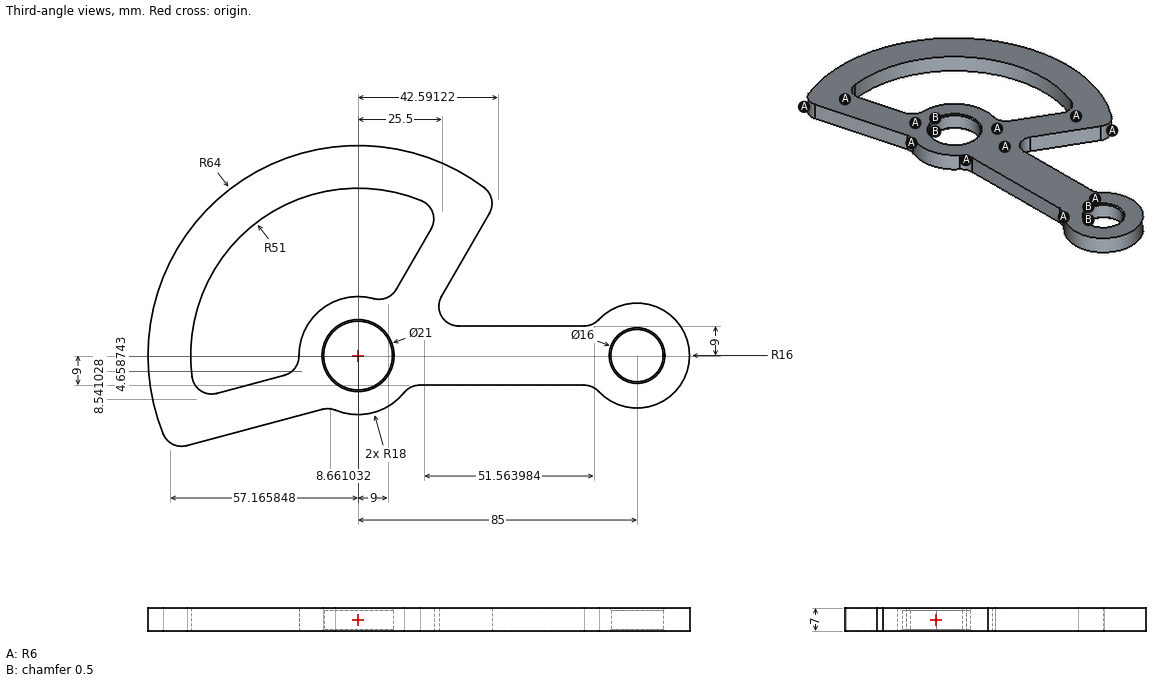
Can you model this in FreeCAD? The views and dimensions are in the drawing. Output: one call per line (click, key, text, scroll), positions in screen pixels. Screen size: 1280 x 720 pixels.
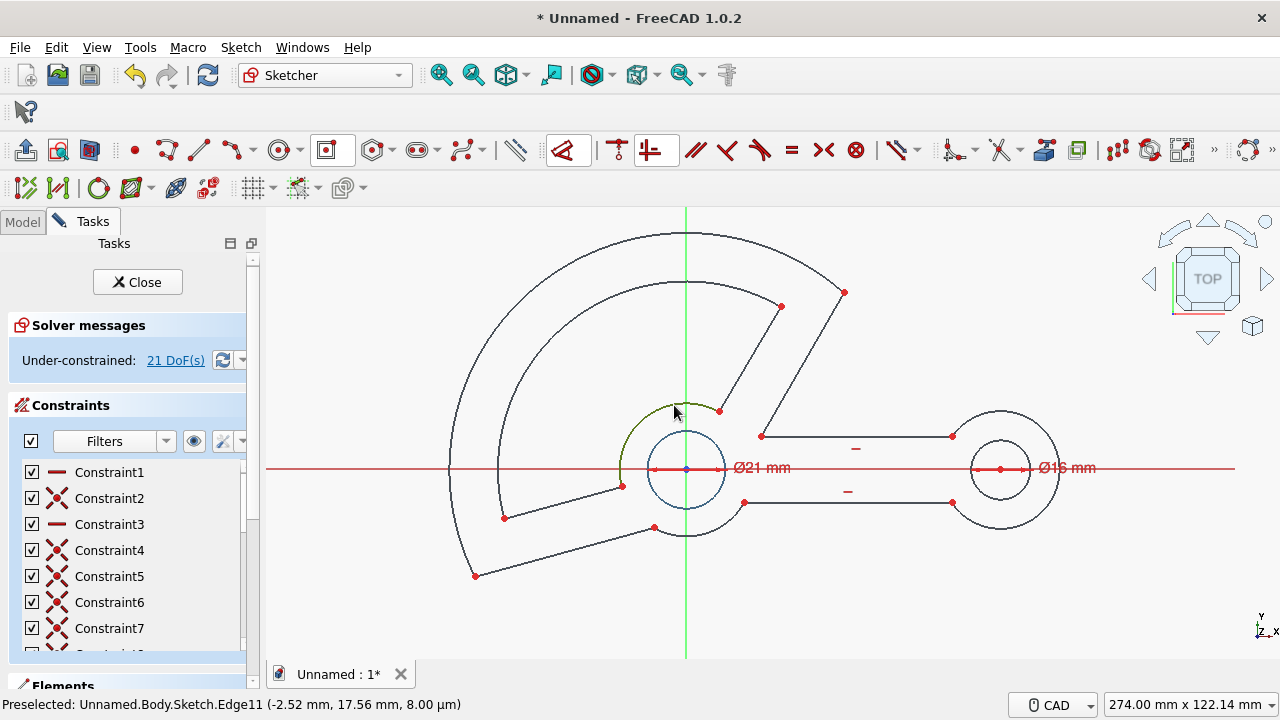
click(618, 150)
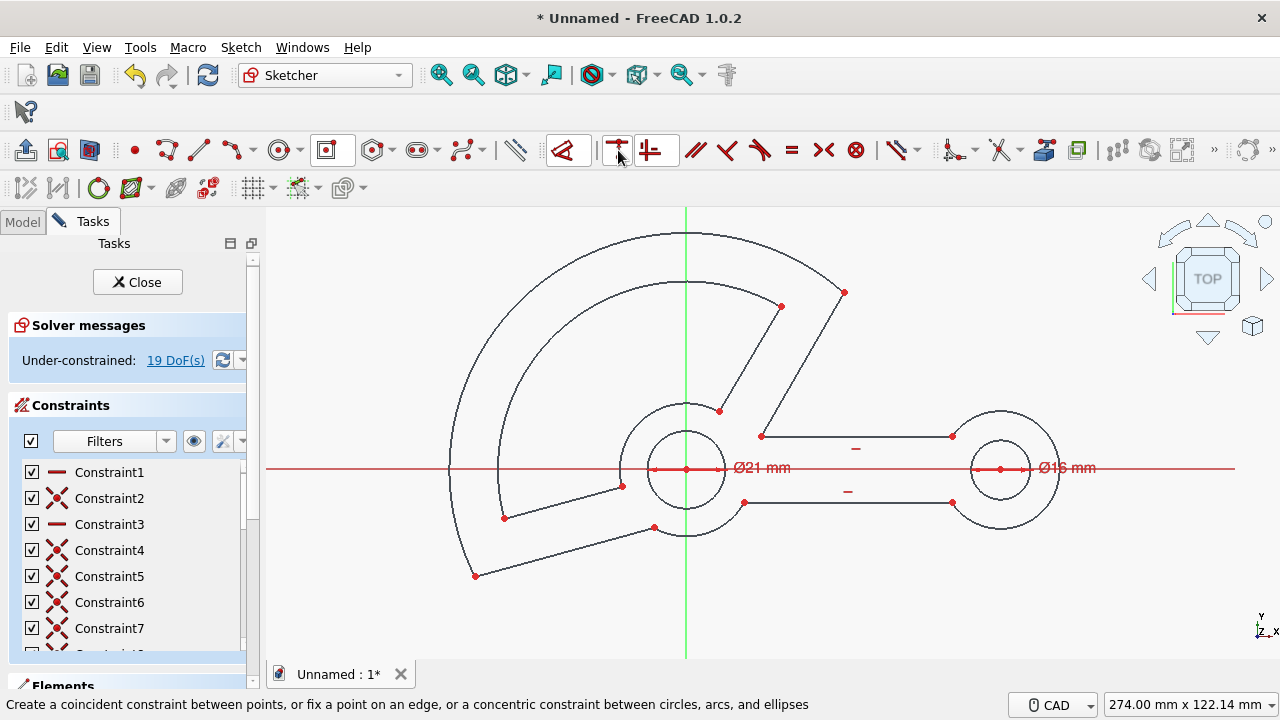
scroll(686, 469, up, 2)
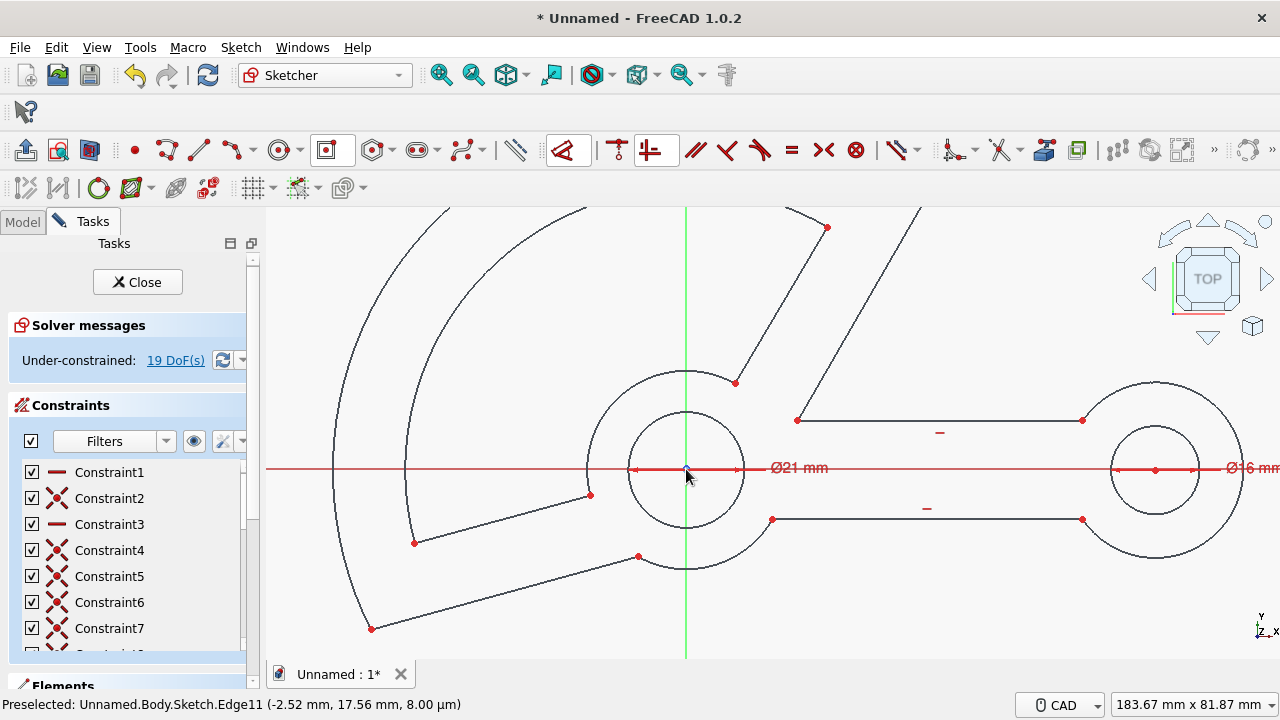
drag(676, 459, 696, 480)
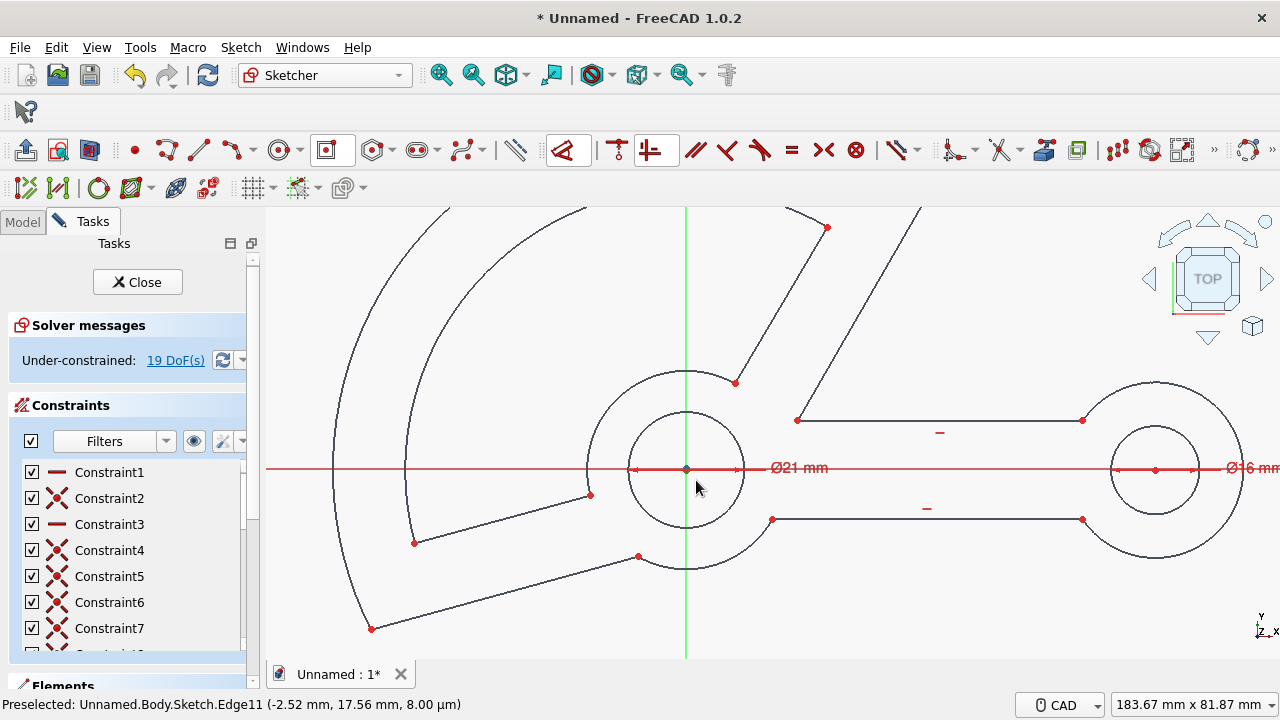
key(c)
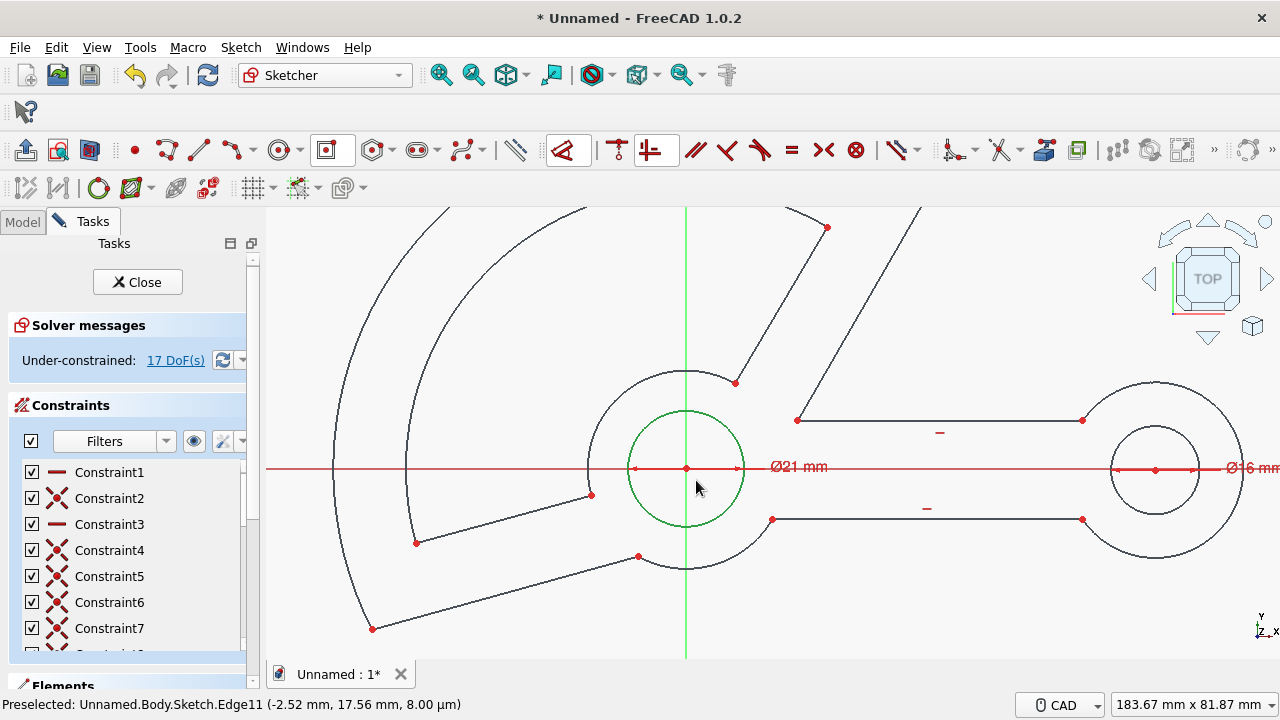
click(682, 569)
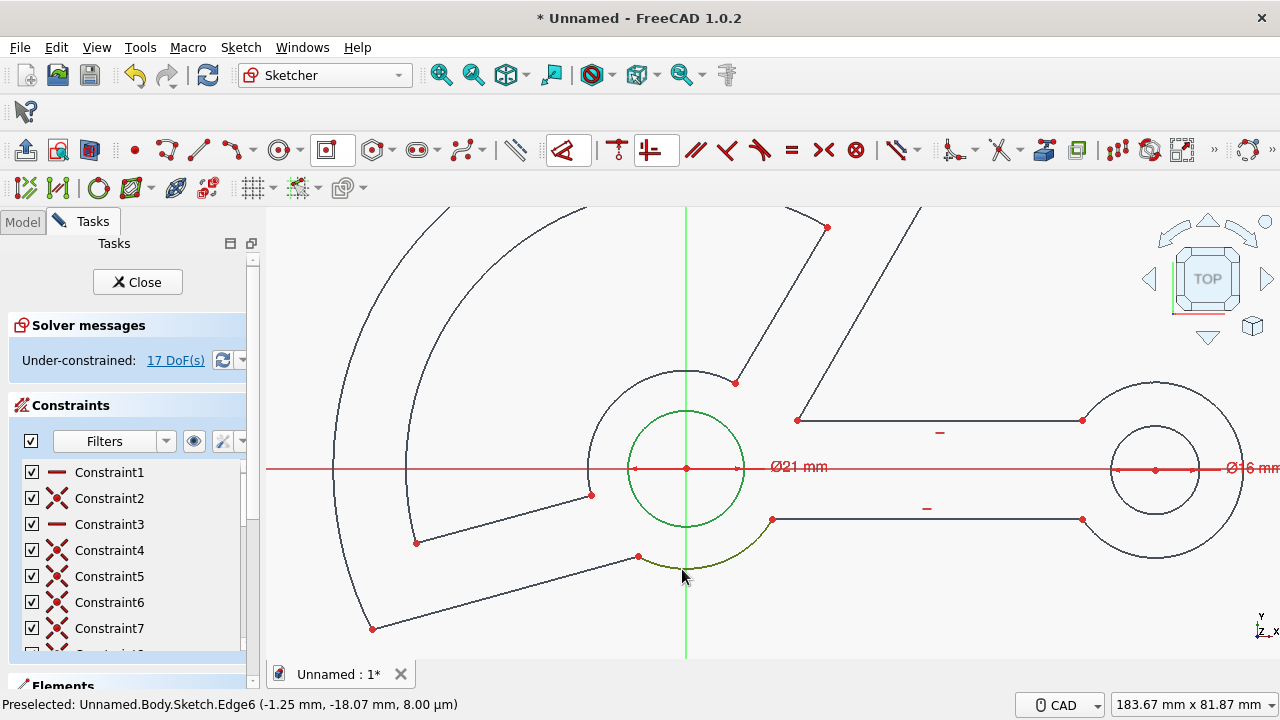
click(668, 372)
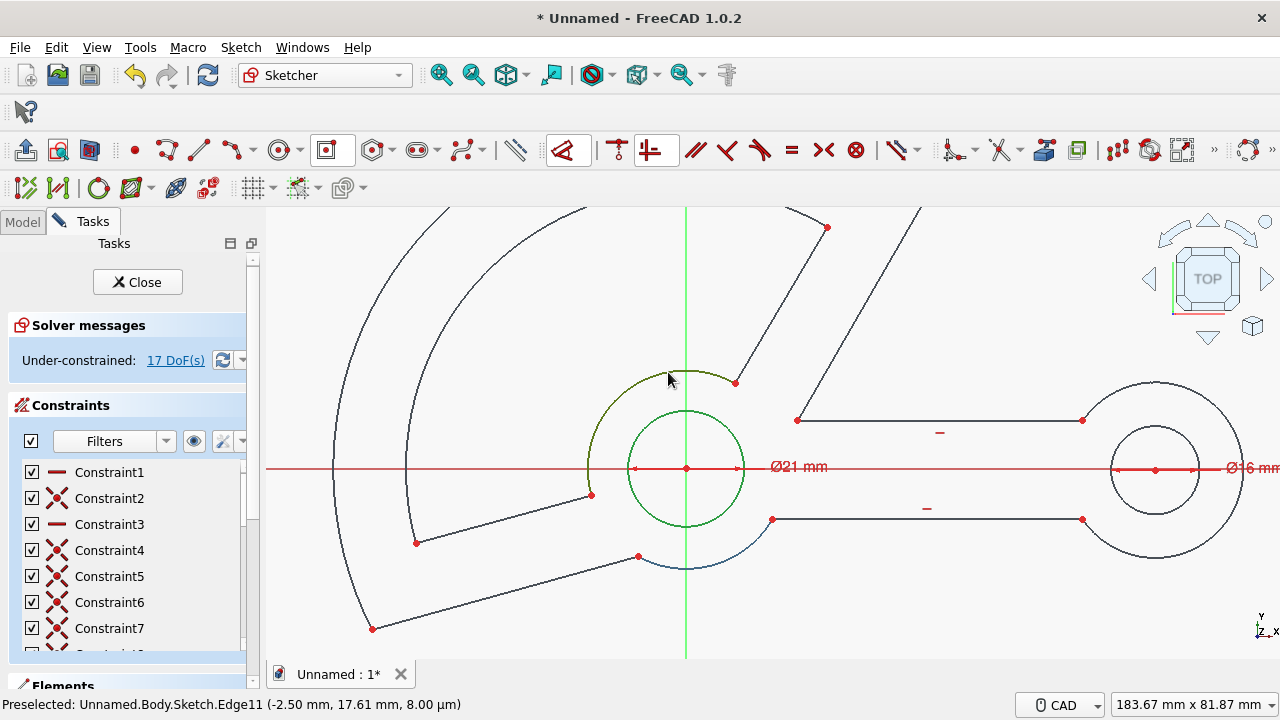
click(792, 150)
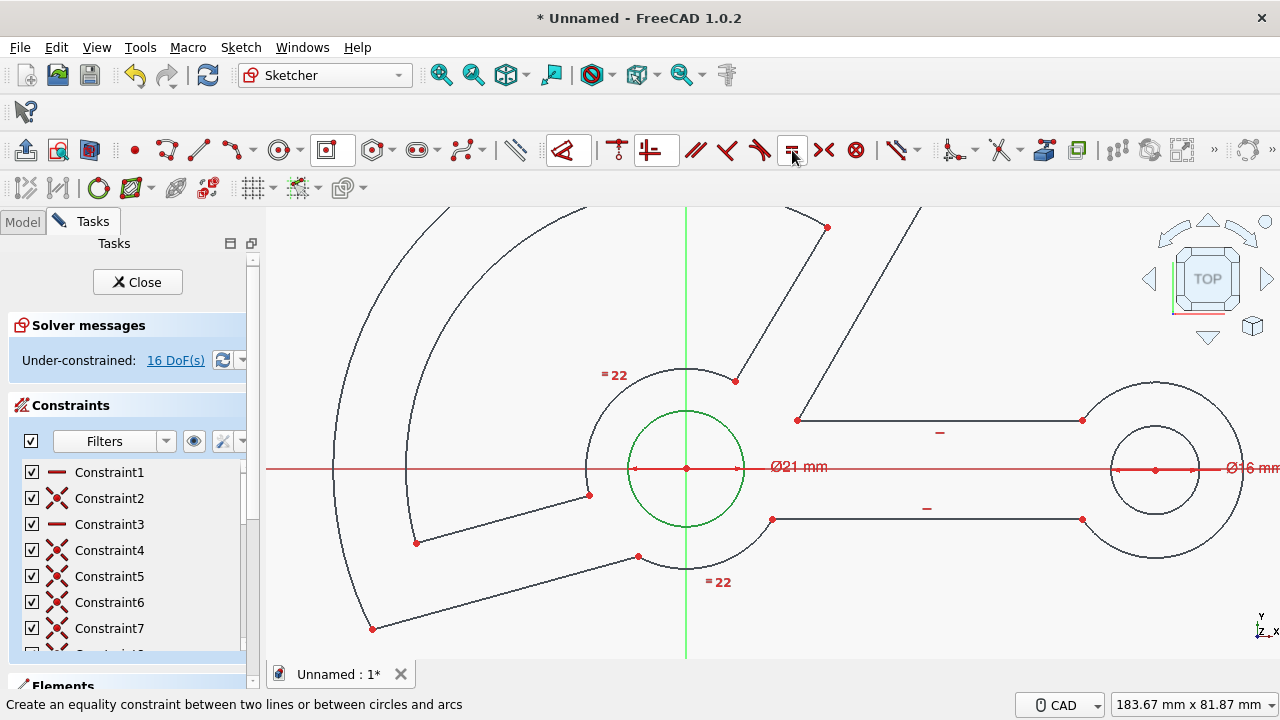
scroll(496, 484, down, 2)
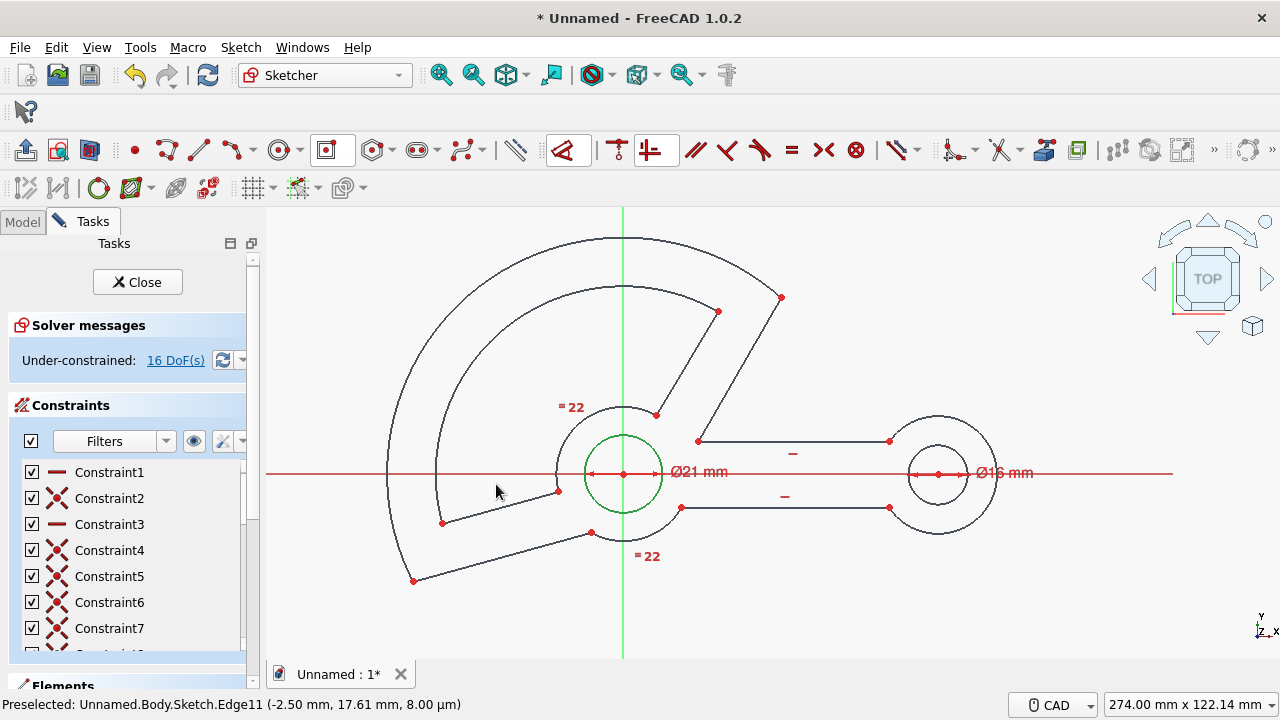
click(938, 475)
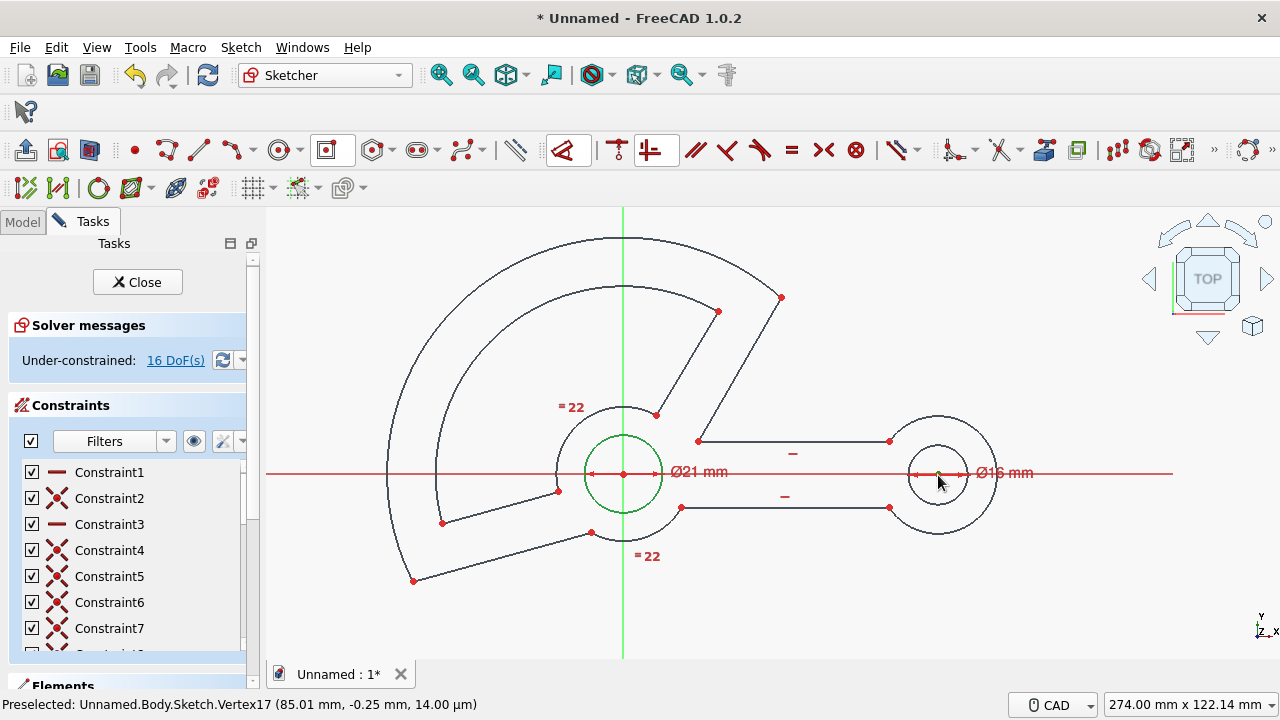
click(353, 474)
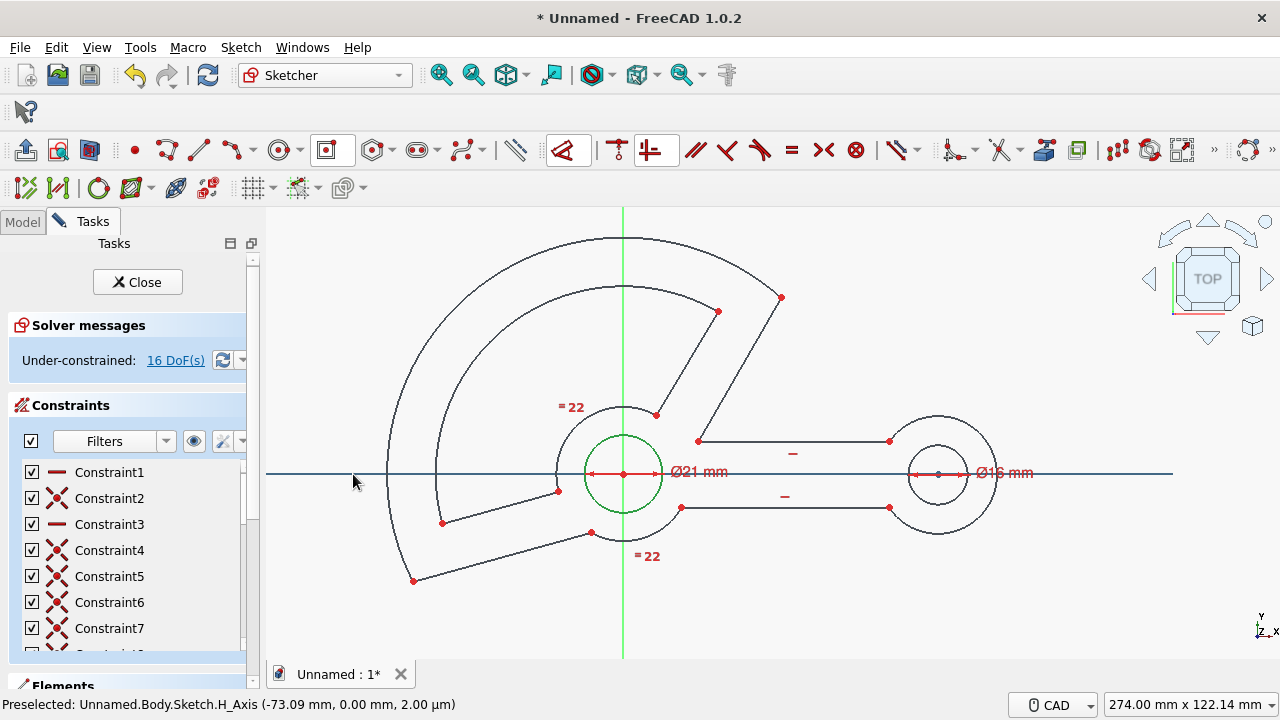
click(618, 150)